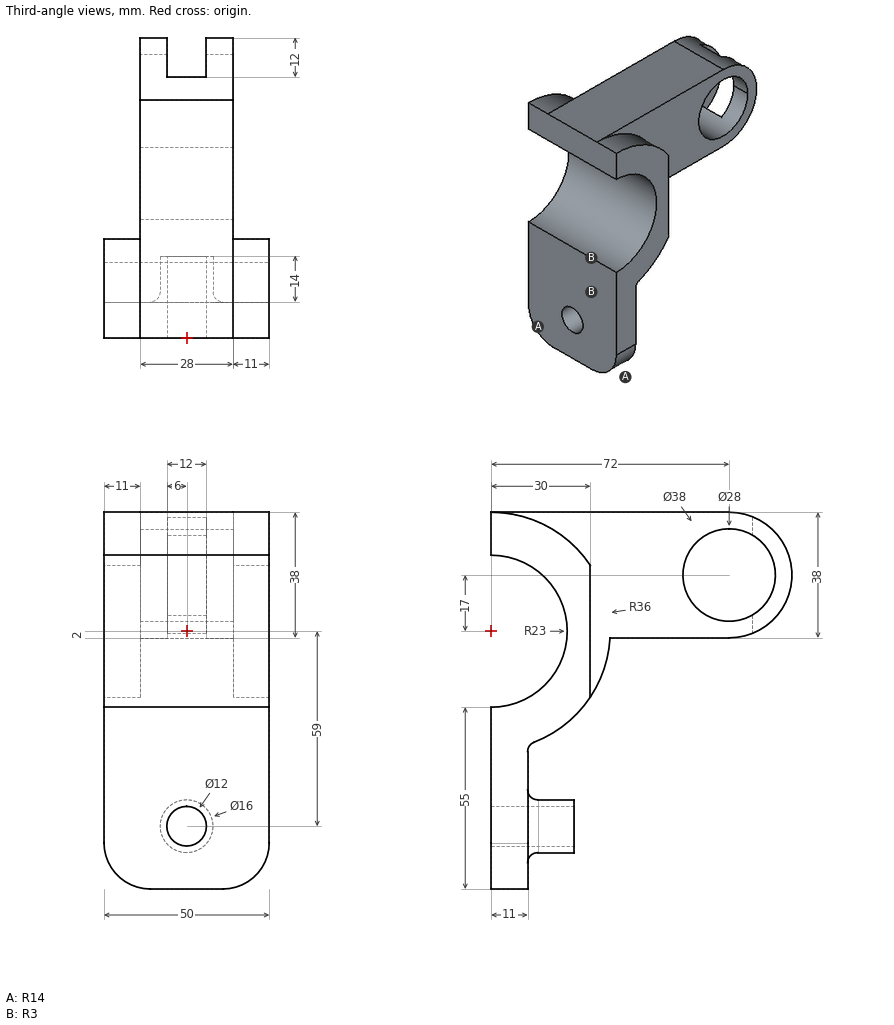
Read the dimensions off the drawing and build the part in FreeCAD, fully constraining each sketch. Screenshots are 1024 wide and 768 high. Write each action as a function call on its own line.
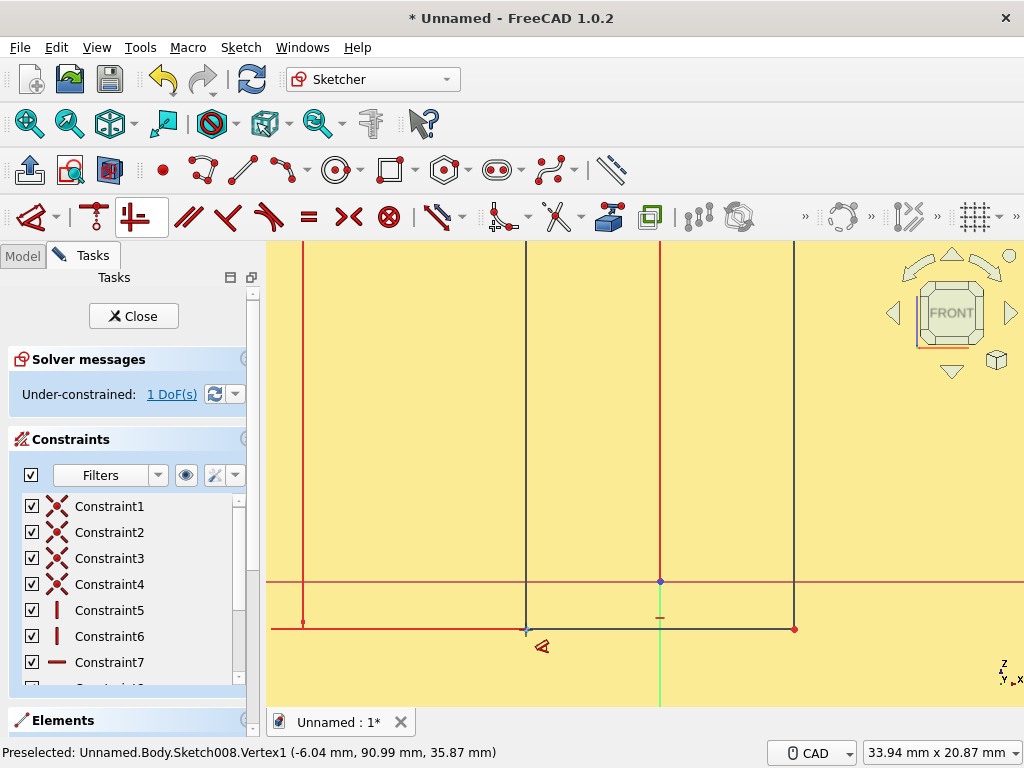
click(526, 629)
click(492, 605)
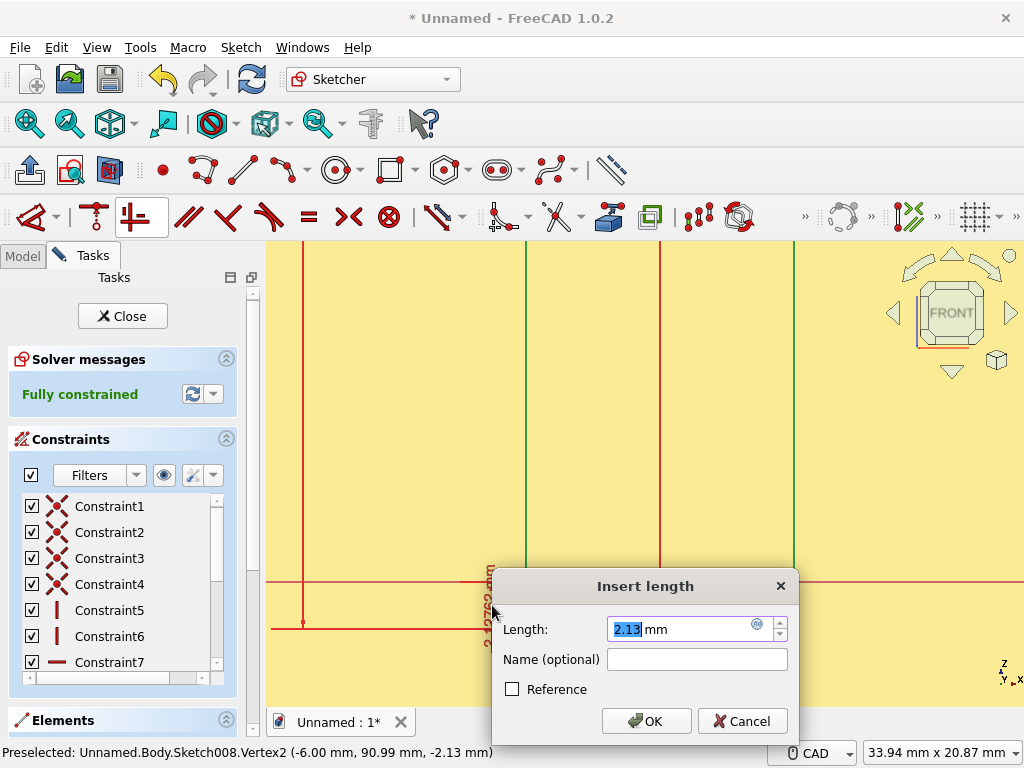
text(2)
key(Return)
key(Escape)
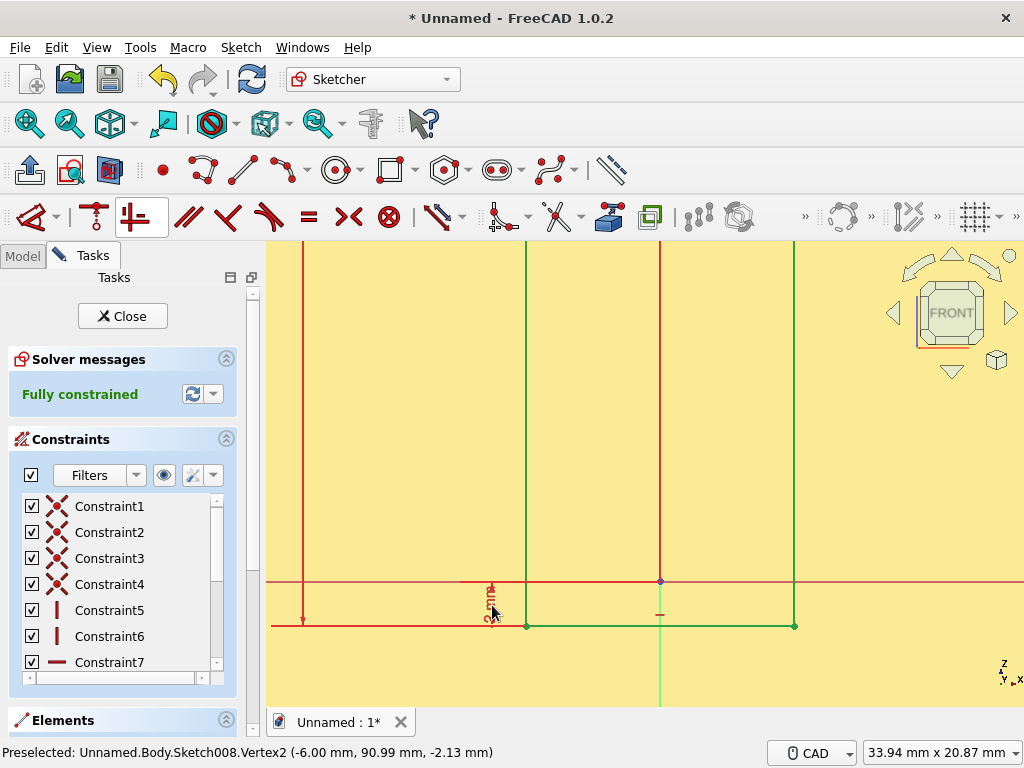
click(123, 316)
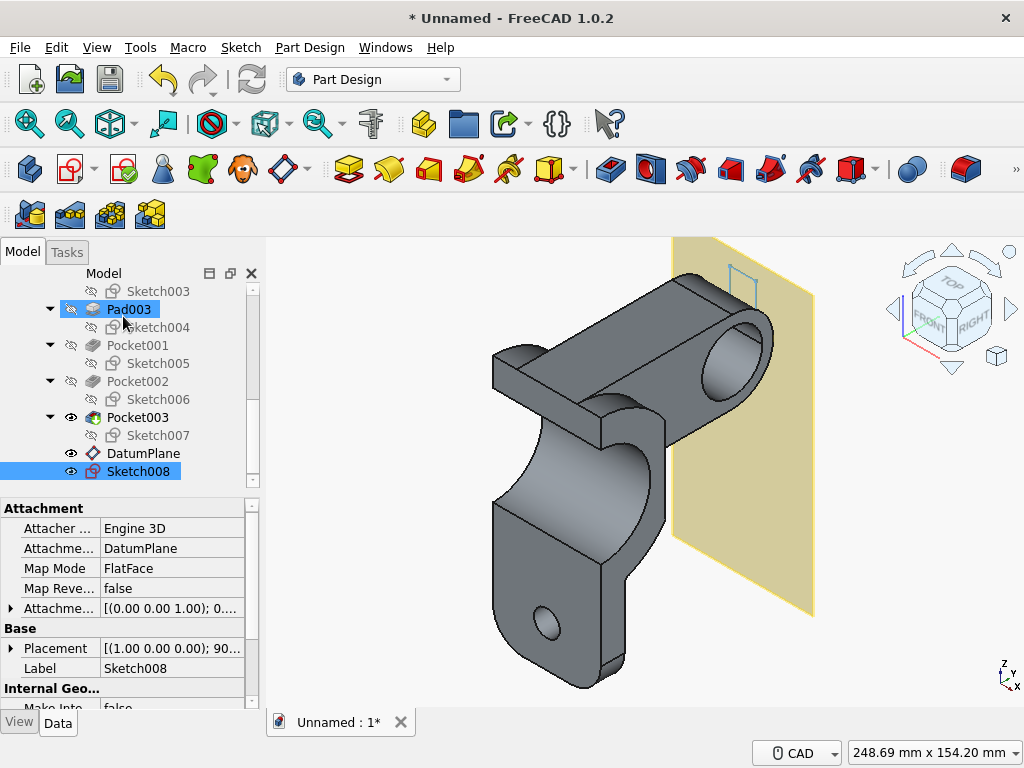
click(612, 170)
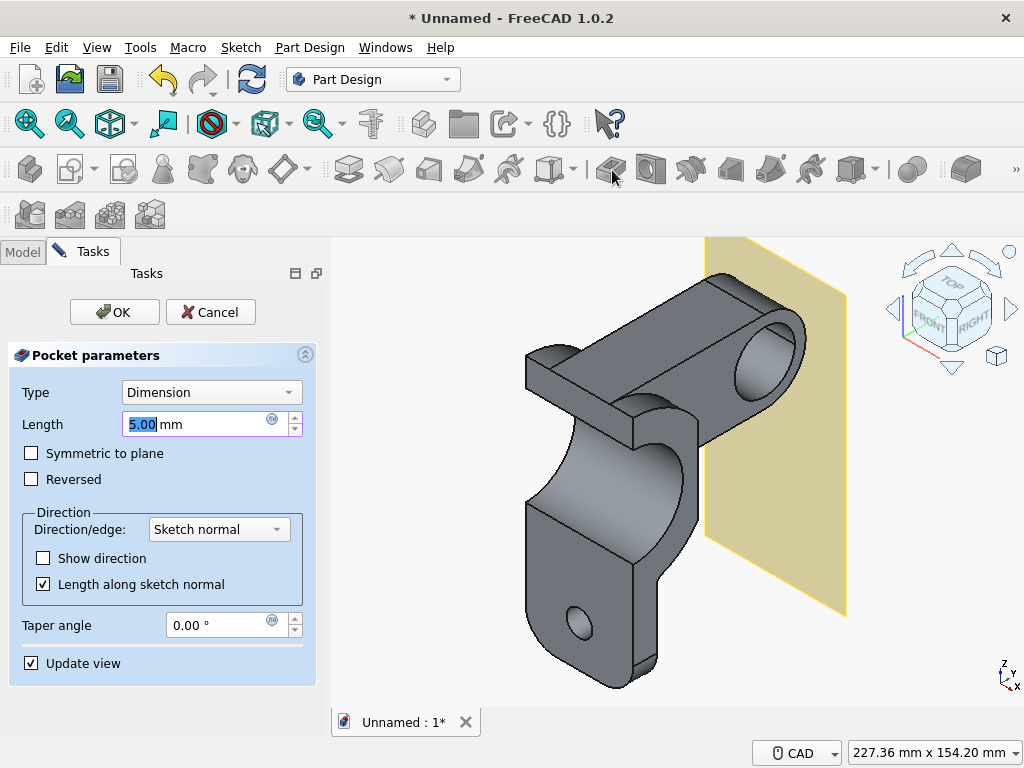
text(12)
key(Tab)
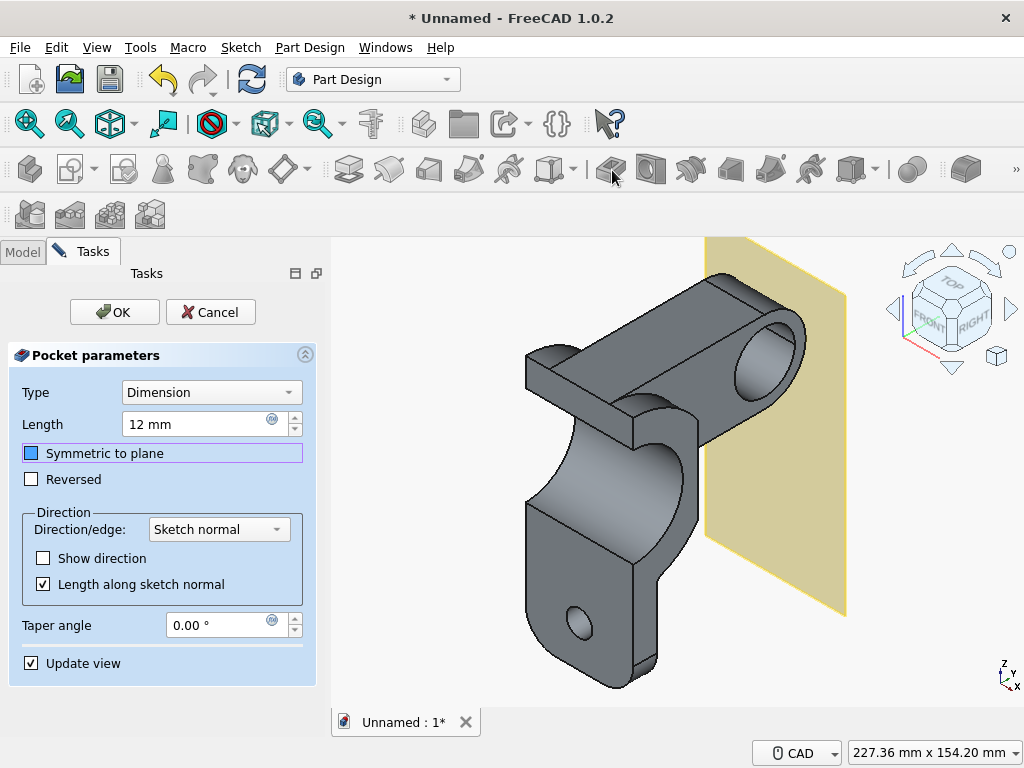
click(30, 479)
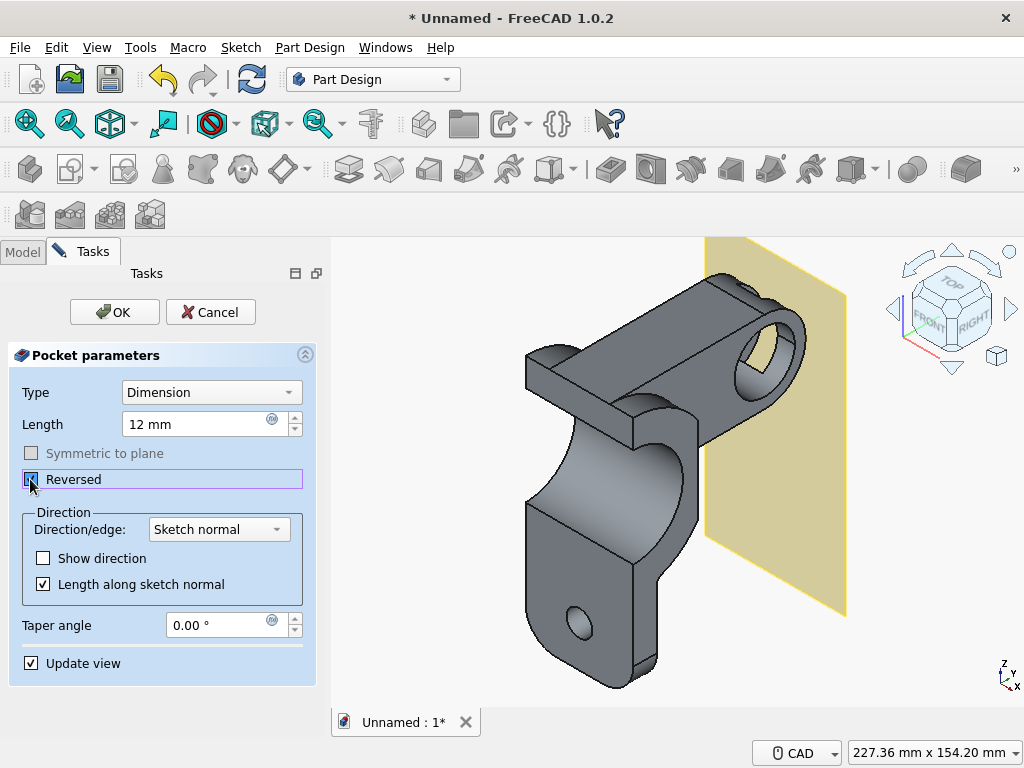
click(115, 312)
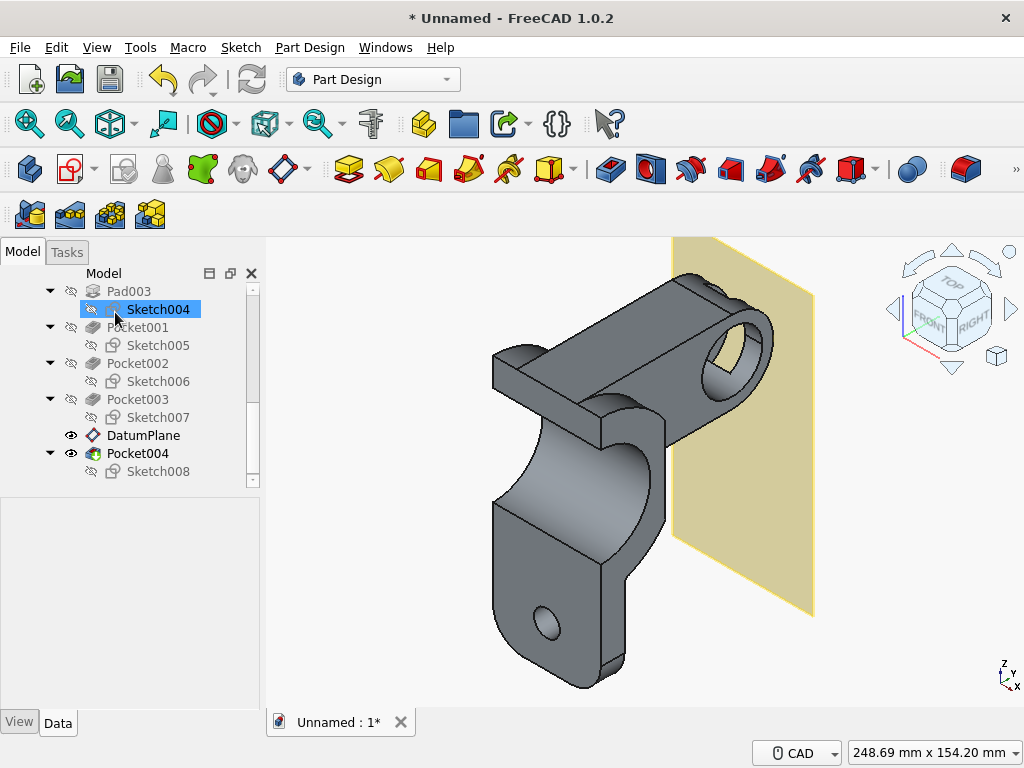
click(116, 435)
key(space)